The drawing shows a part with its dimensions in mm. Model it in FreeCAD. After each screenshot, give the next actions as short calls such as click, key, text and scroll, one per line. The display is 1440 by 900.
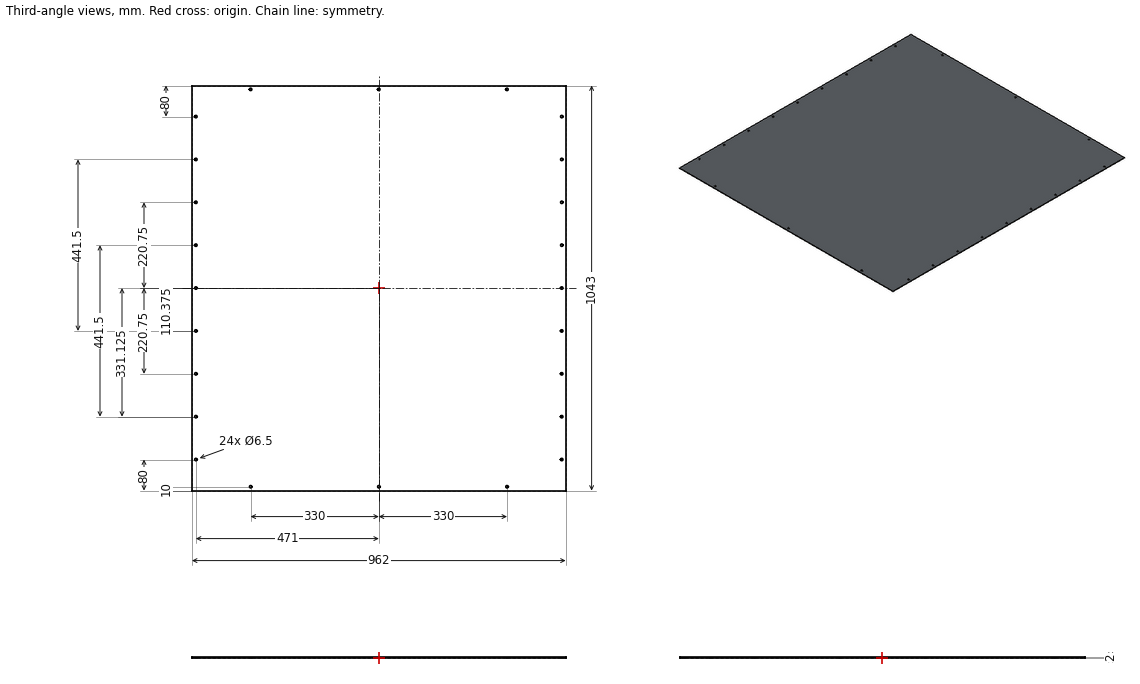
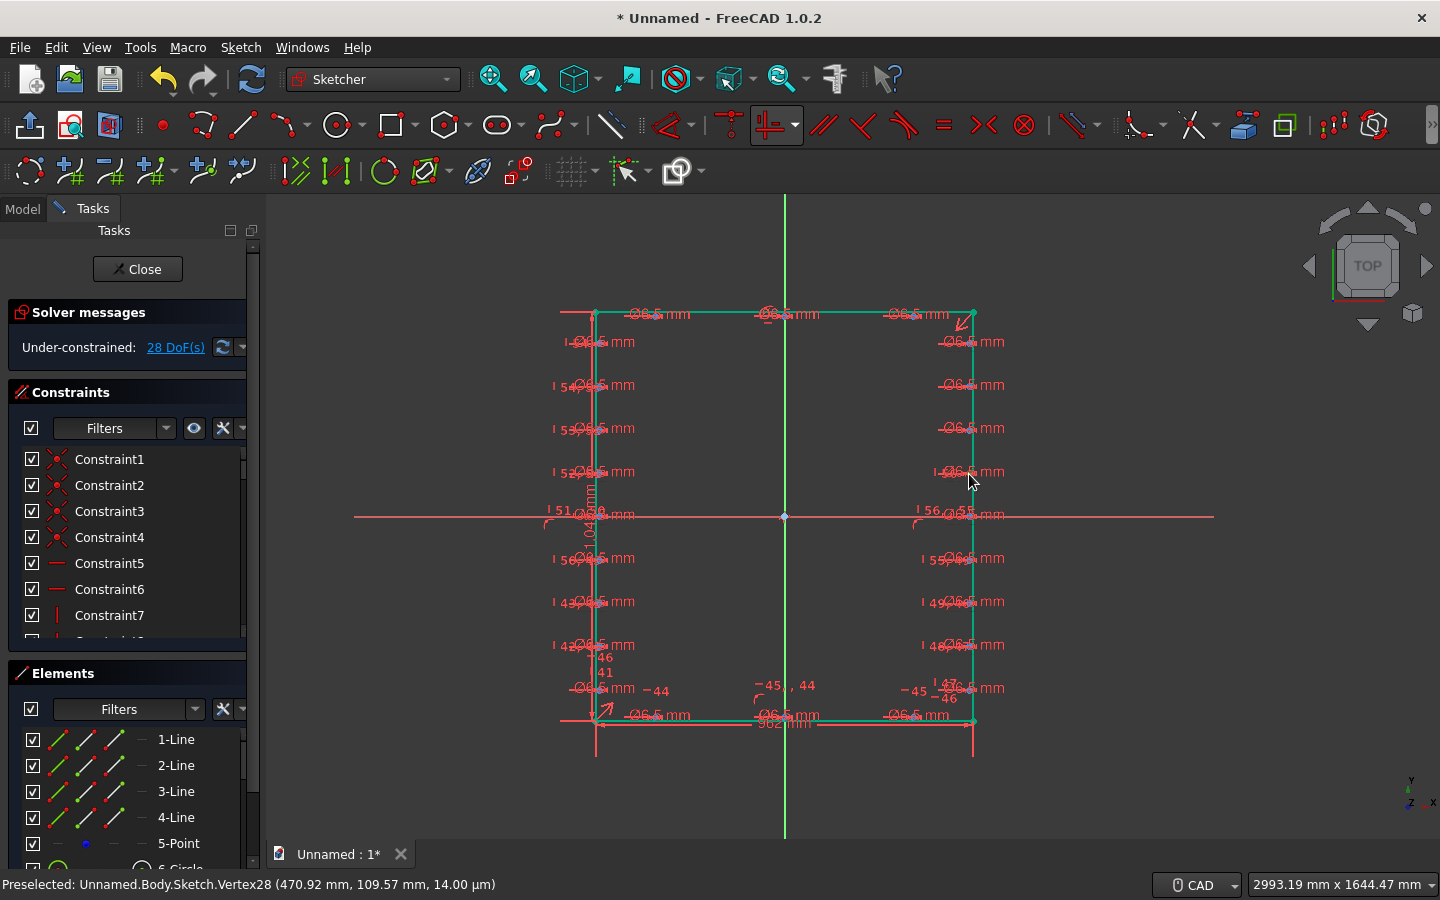
click(969, 430)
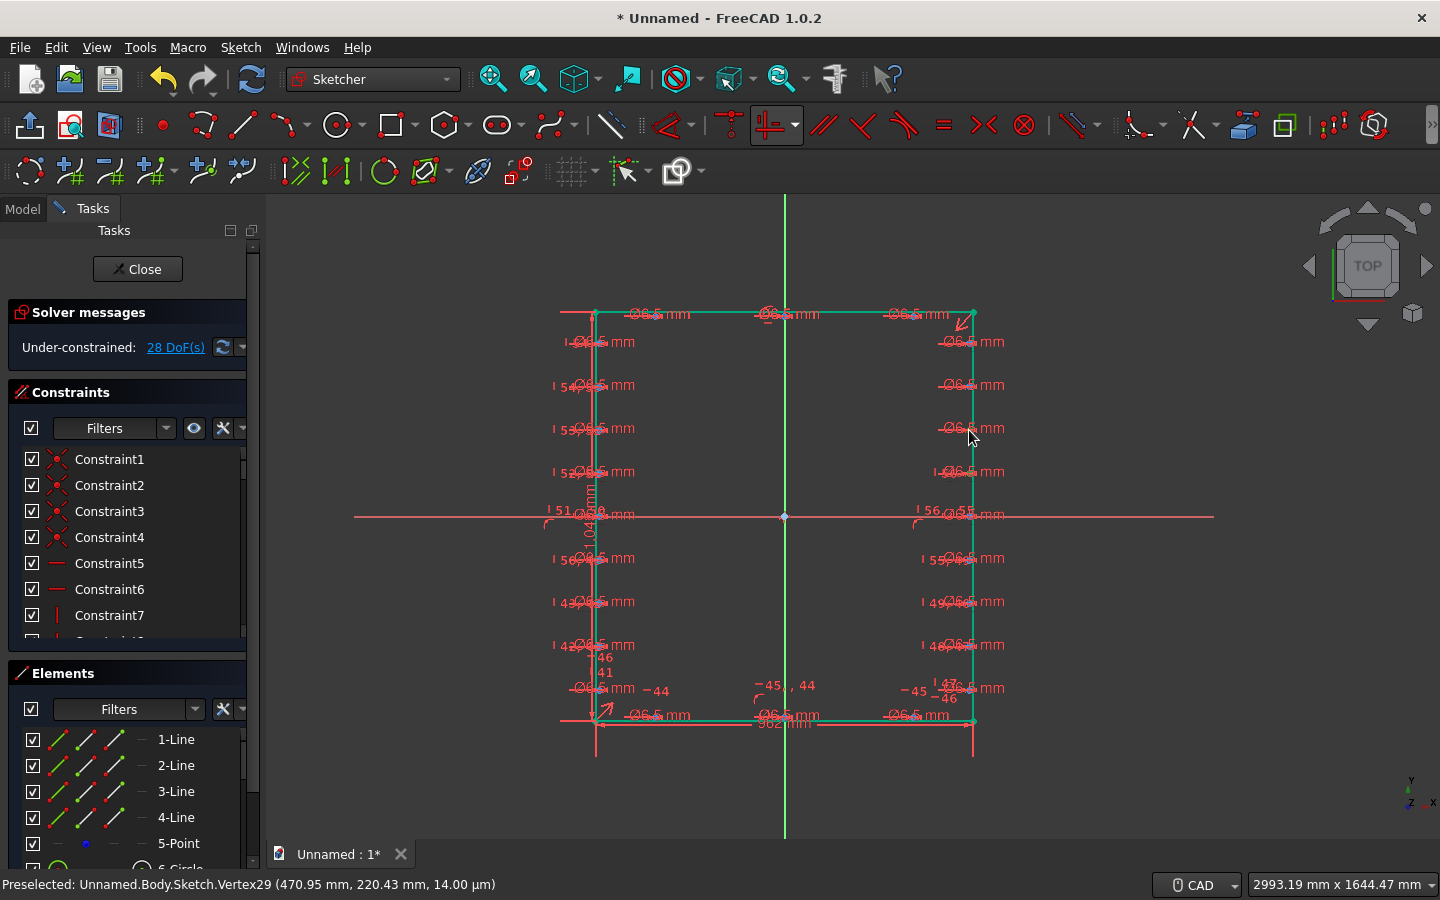
click(798, 126)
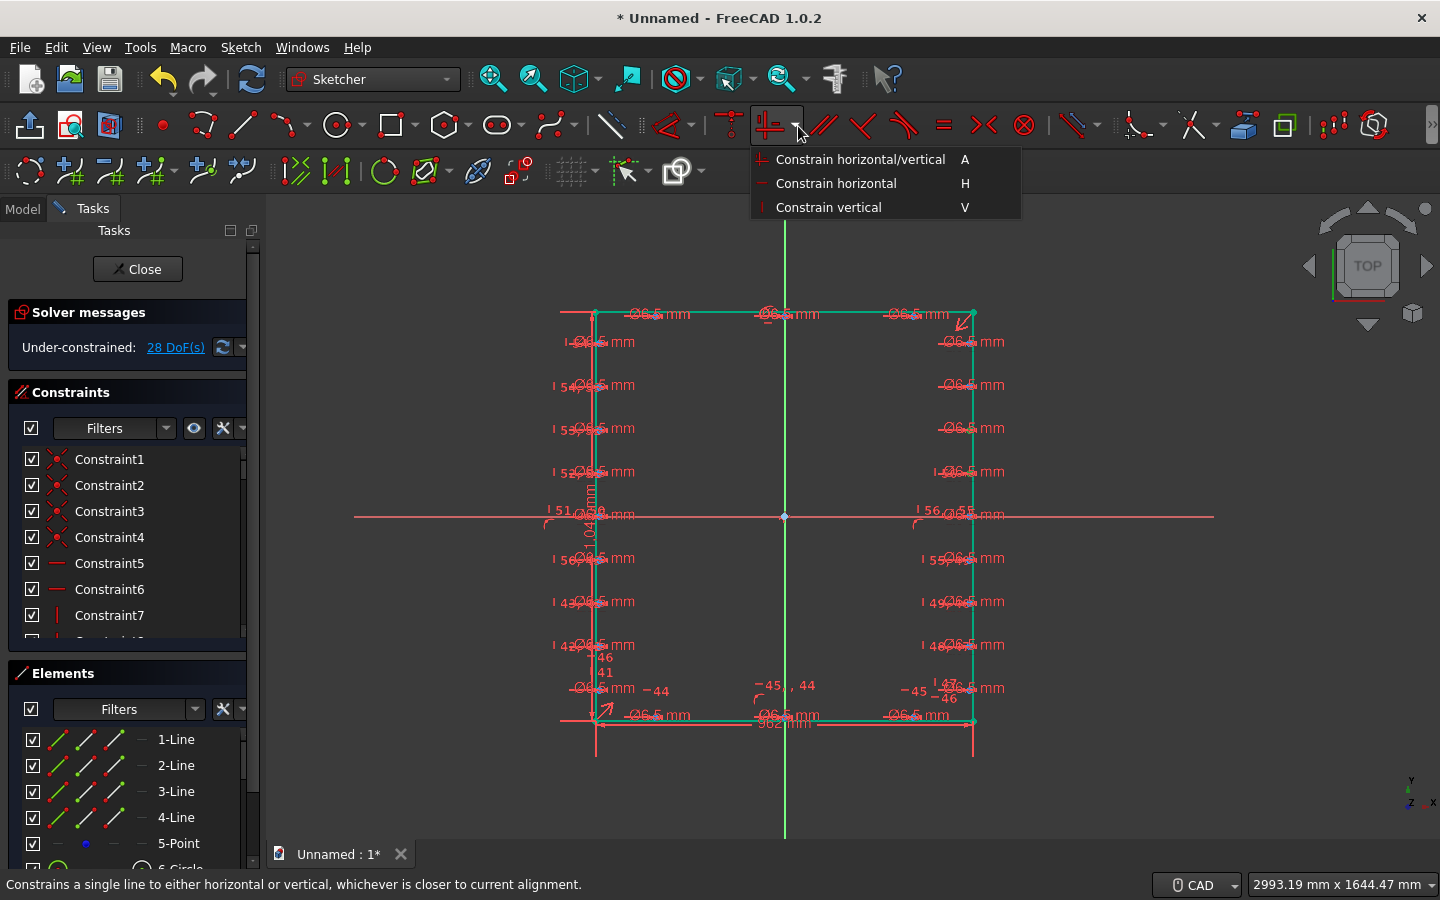
click(886, 207)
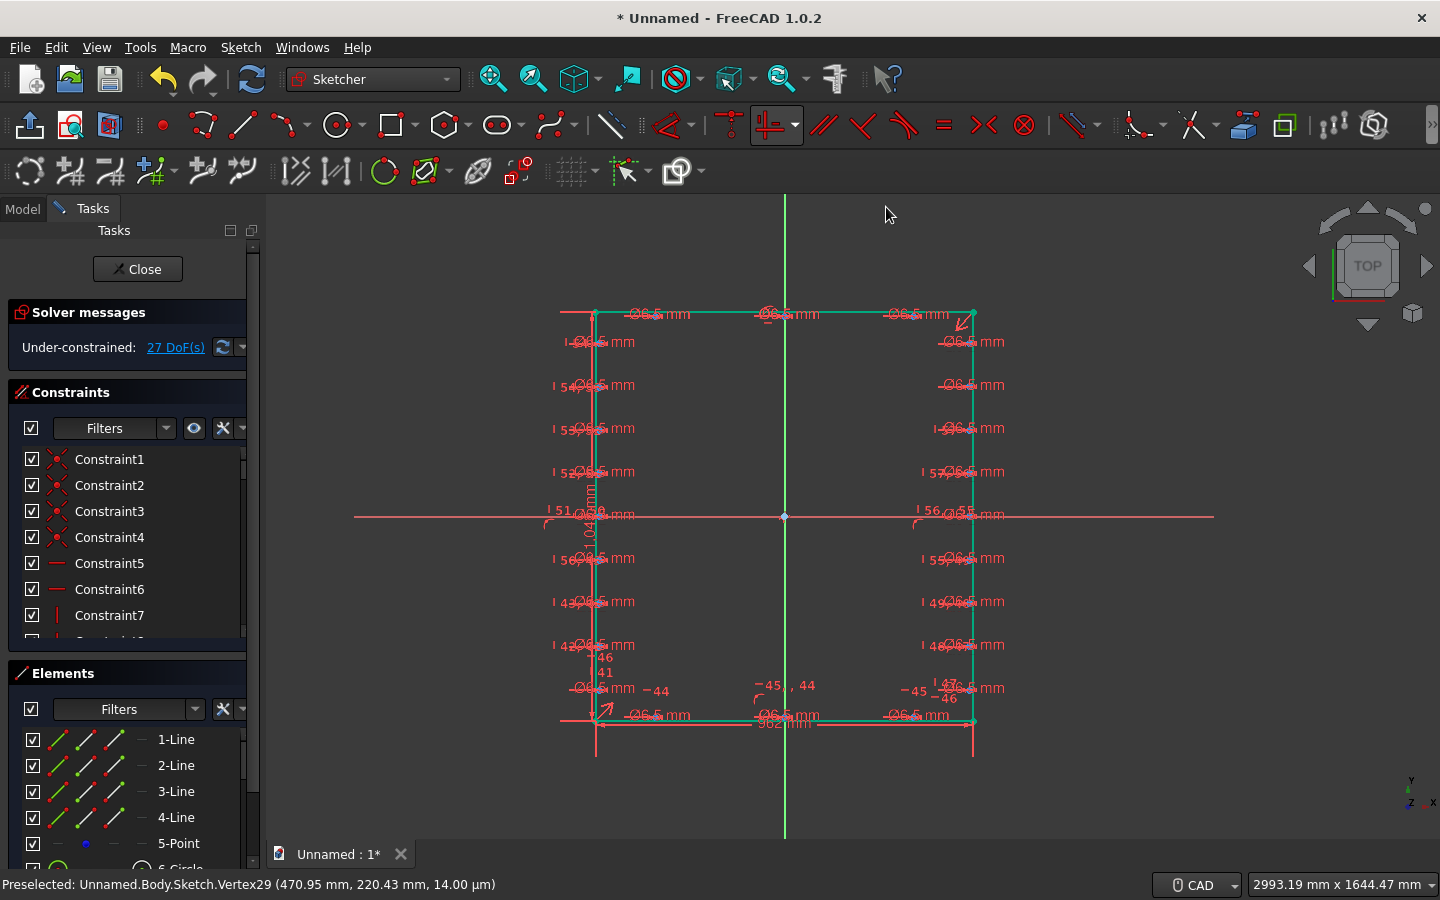
click(655, 316)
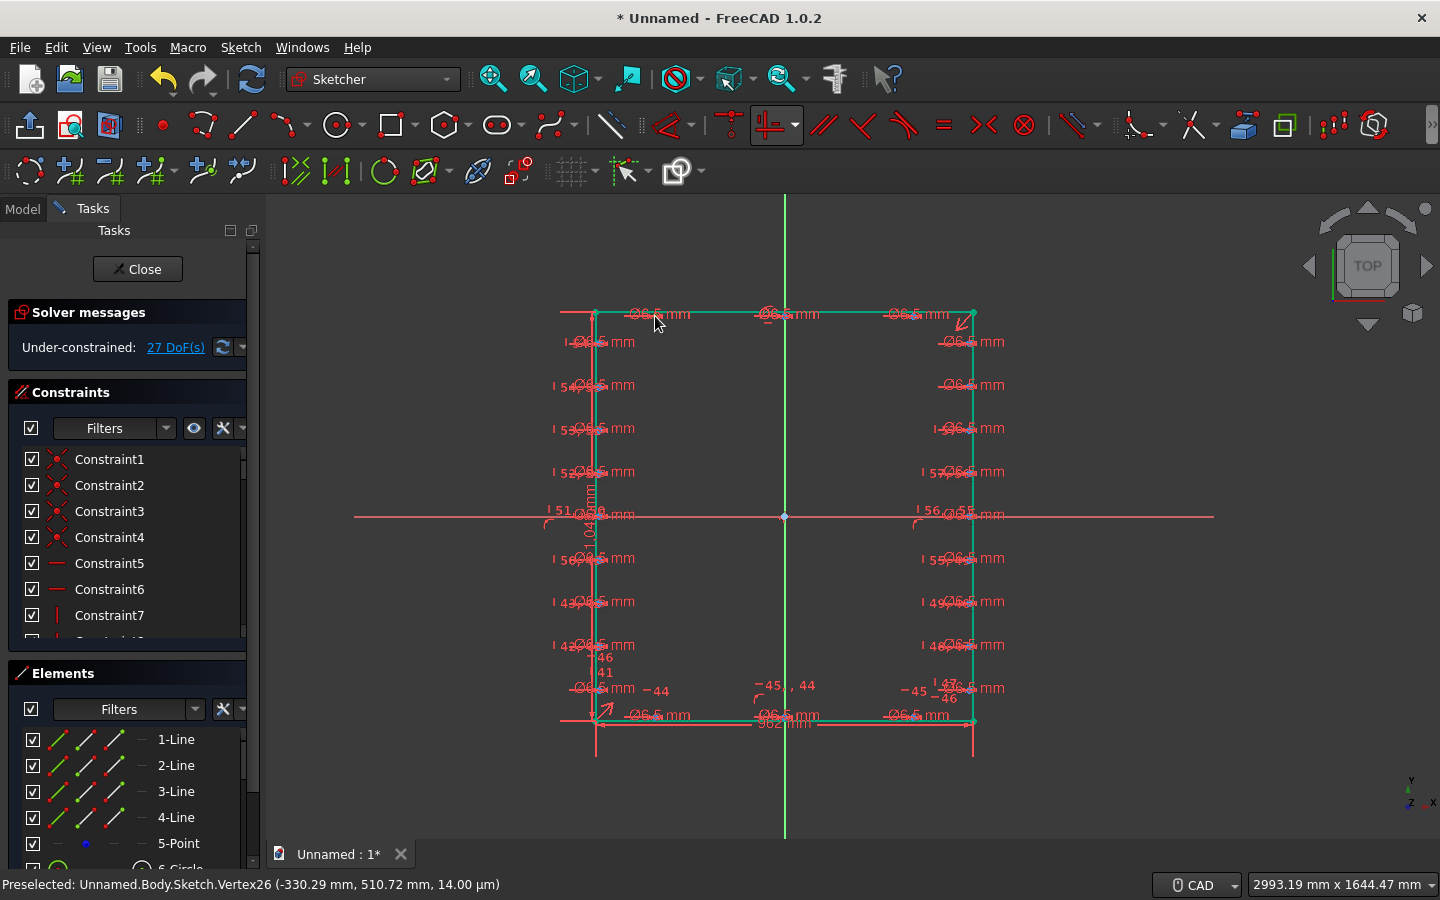
click(785, 316)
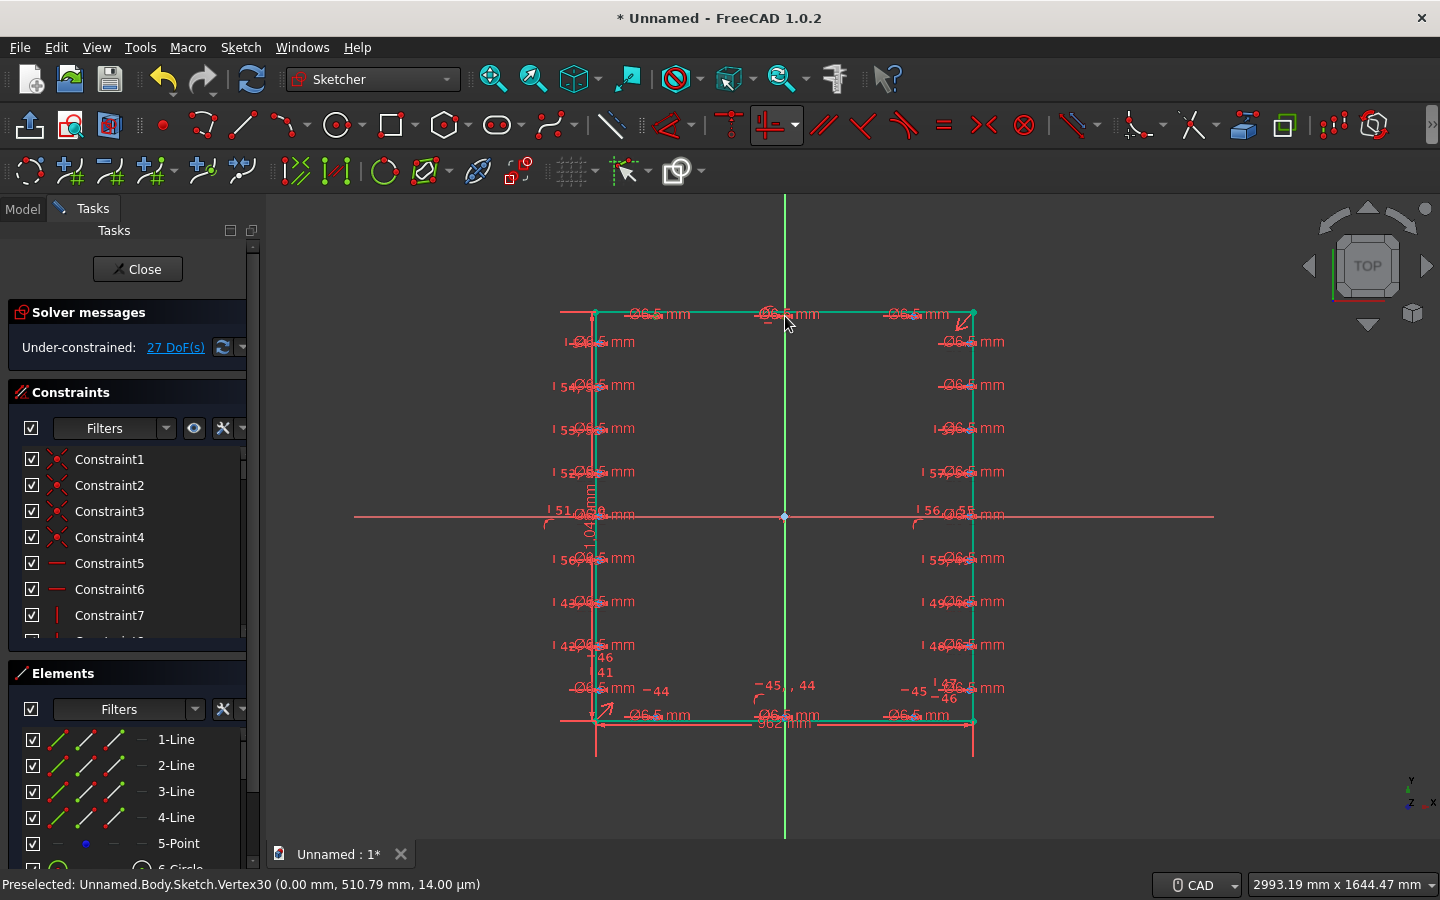
click(798, 126)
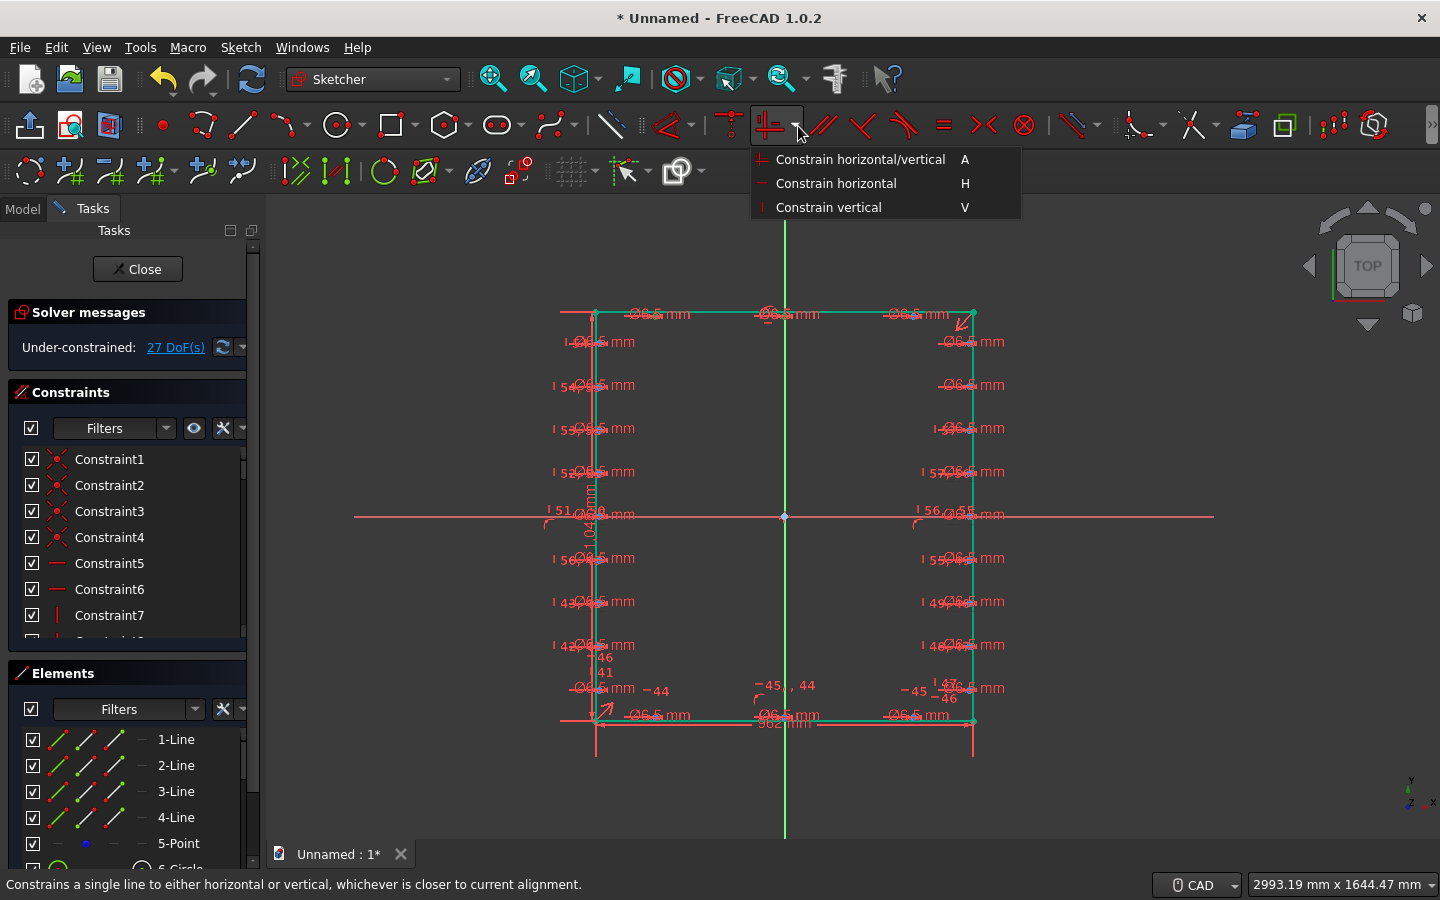
click(886, 183)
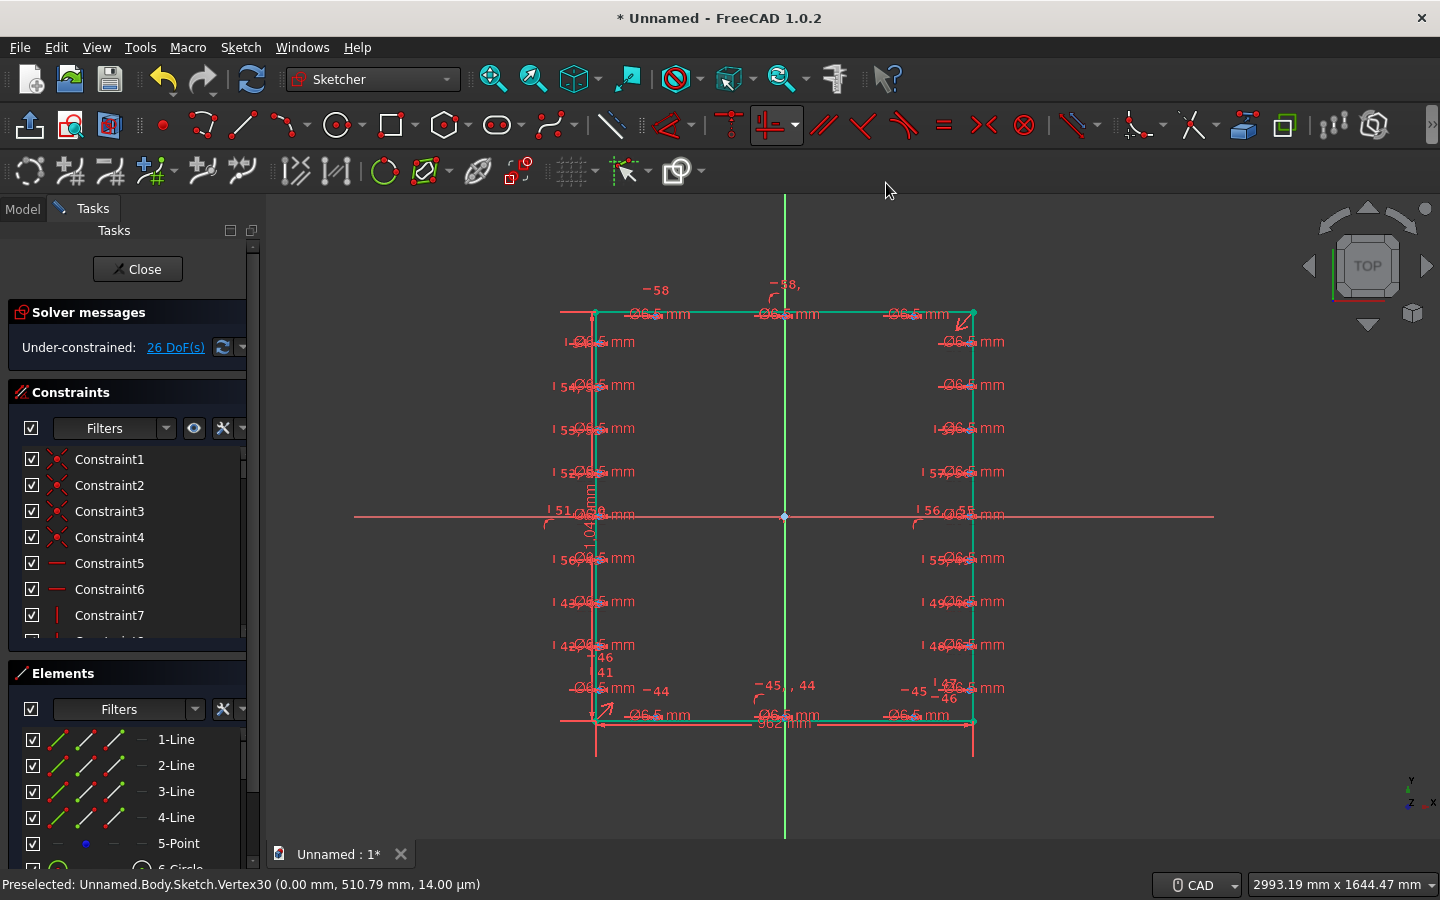
click(969, 430)